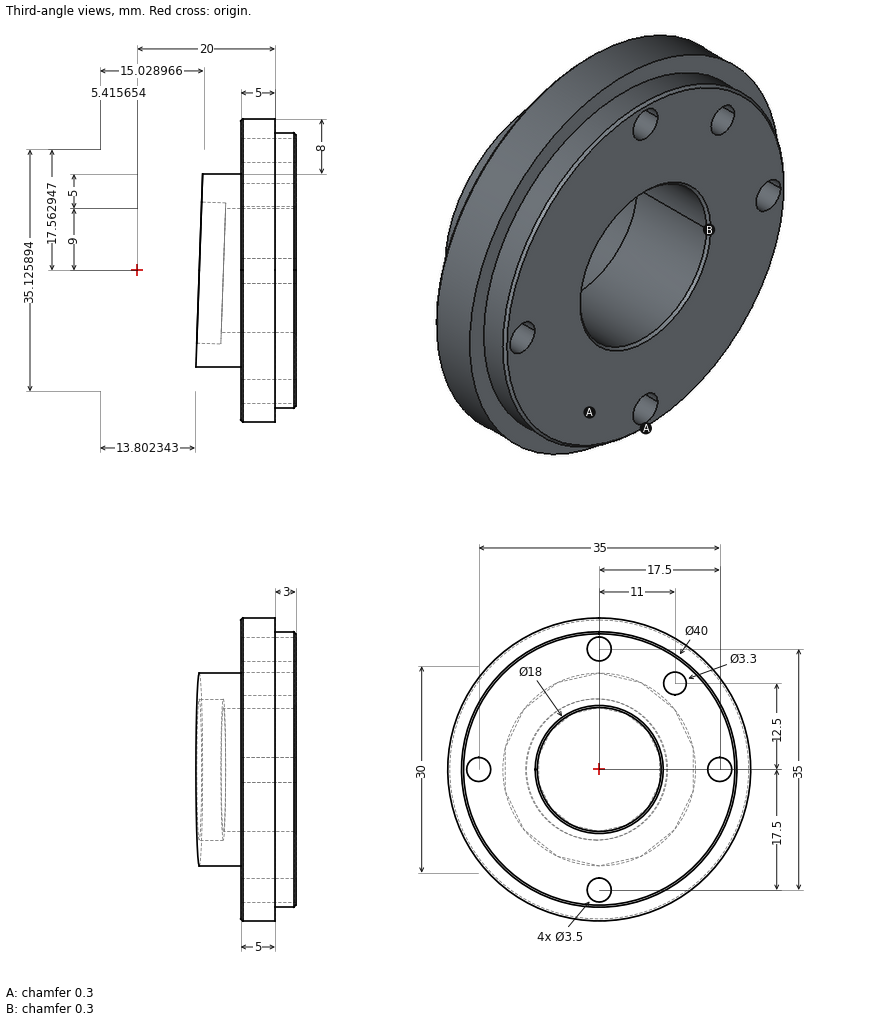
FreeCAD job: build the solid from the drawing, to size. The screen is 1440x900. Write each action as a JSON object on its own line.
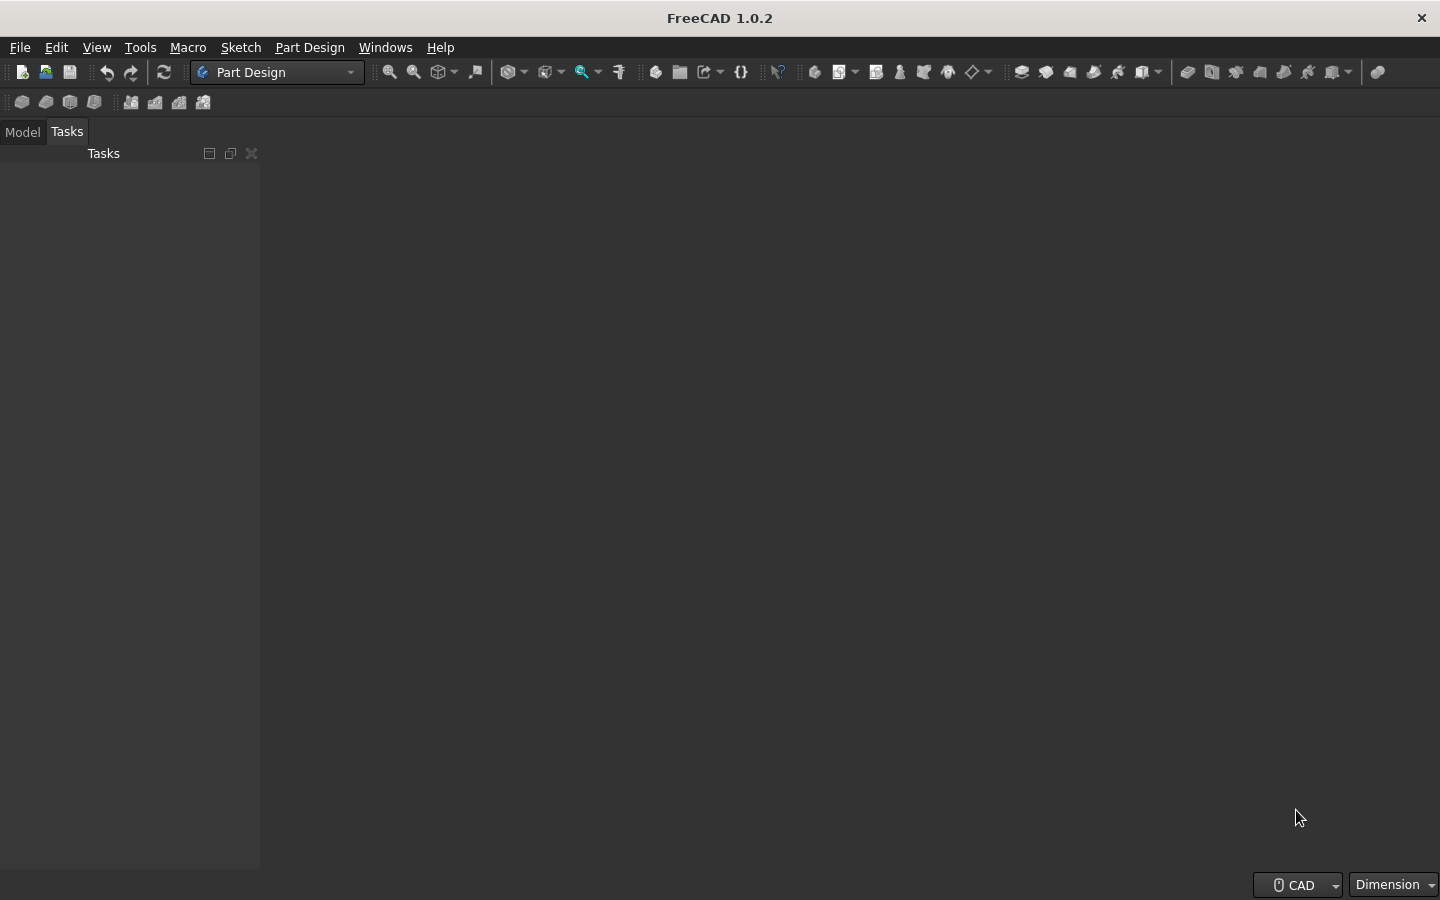
{"action": "left_click", "coordinate": [22, 72]}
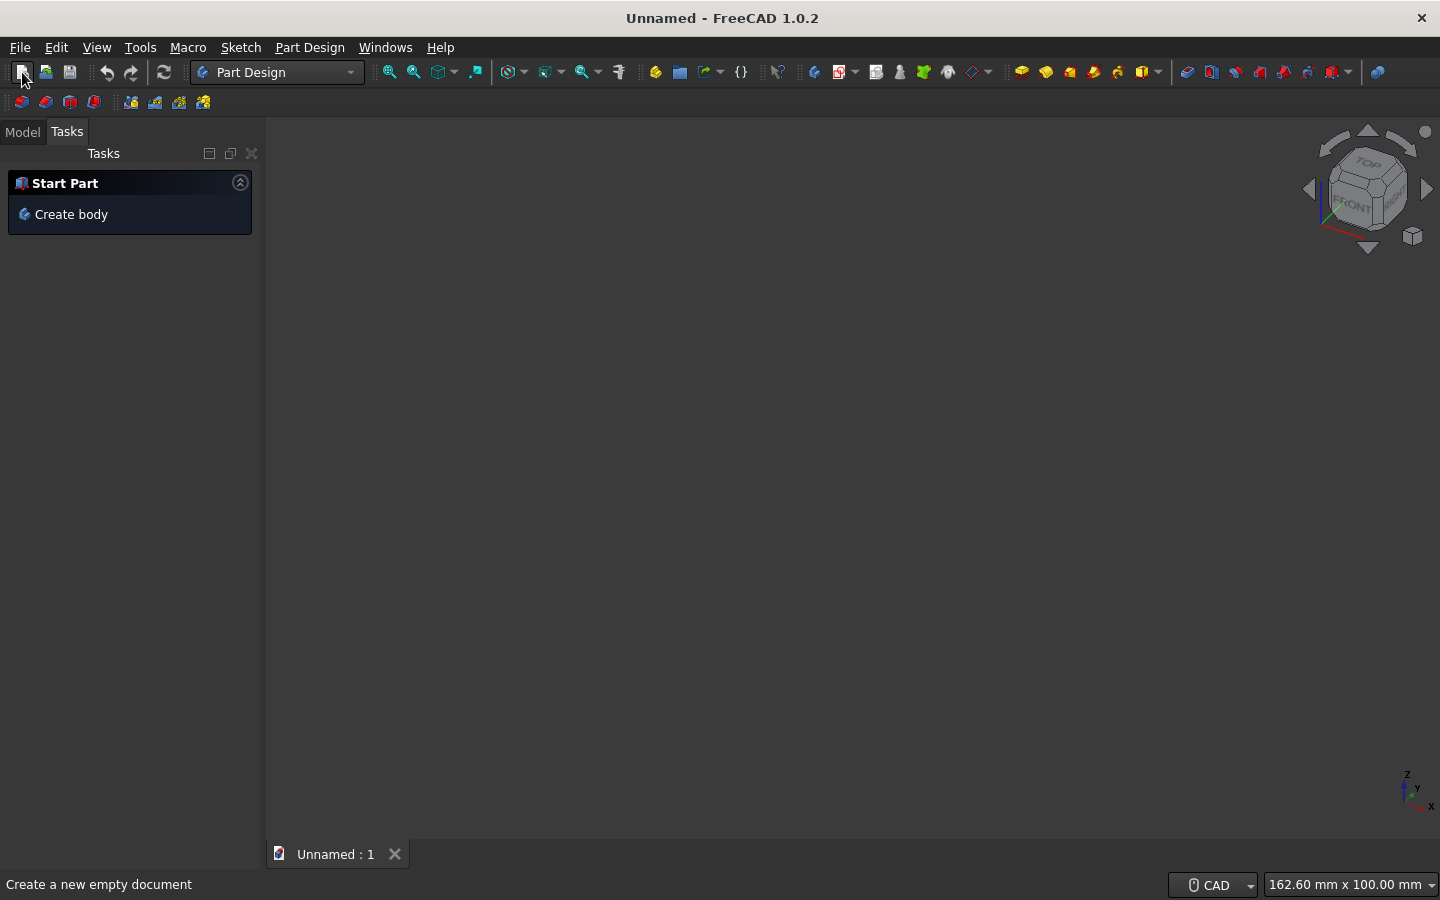
{"action": "left_click", "coordinate": [840, 72]}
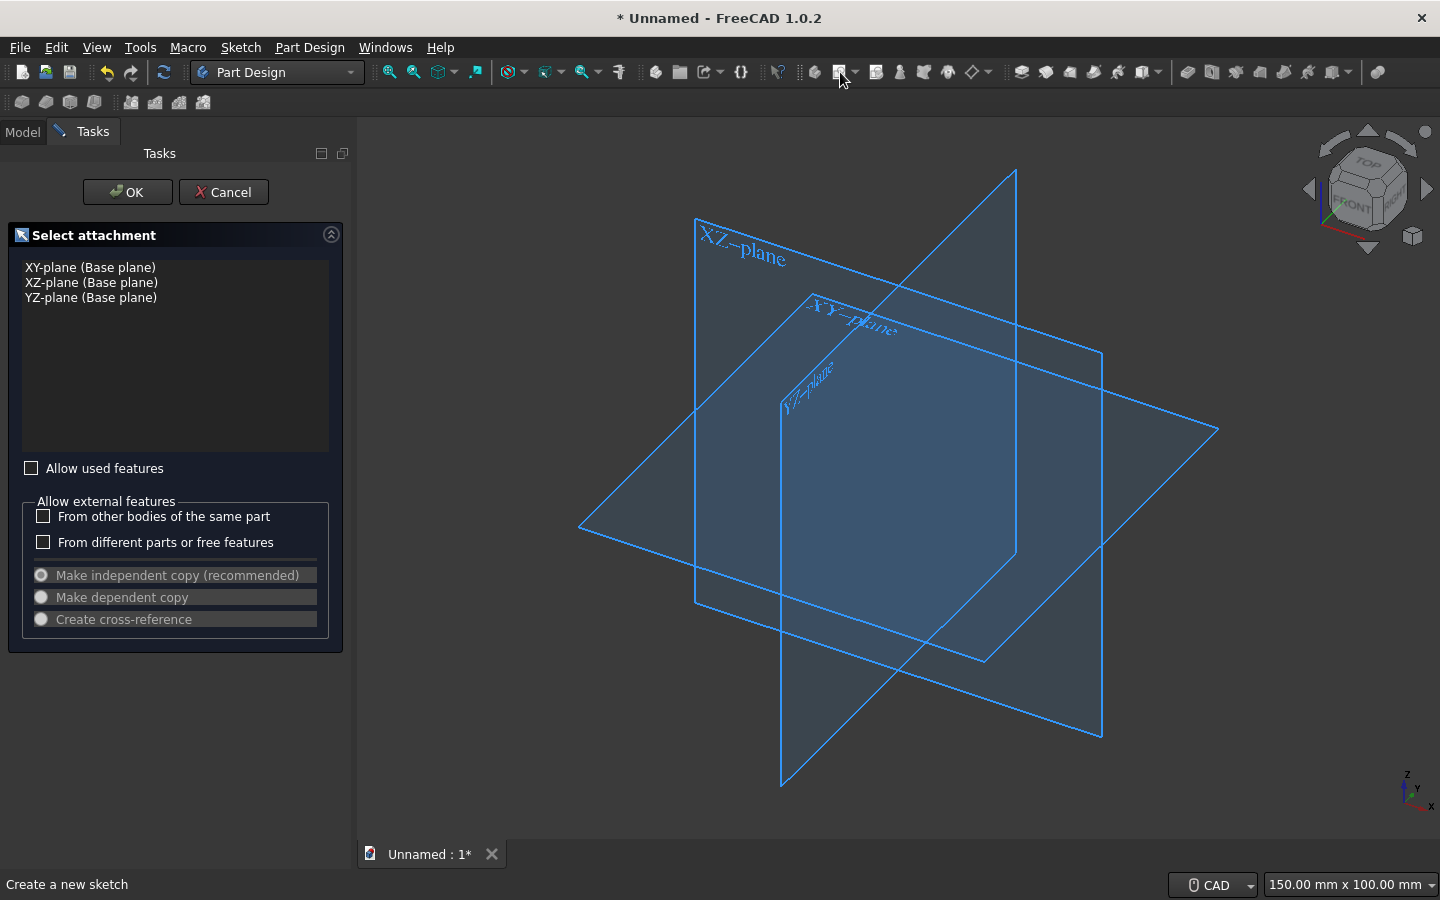
{"action": "left_click", "coordinate": [82, 268]}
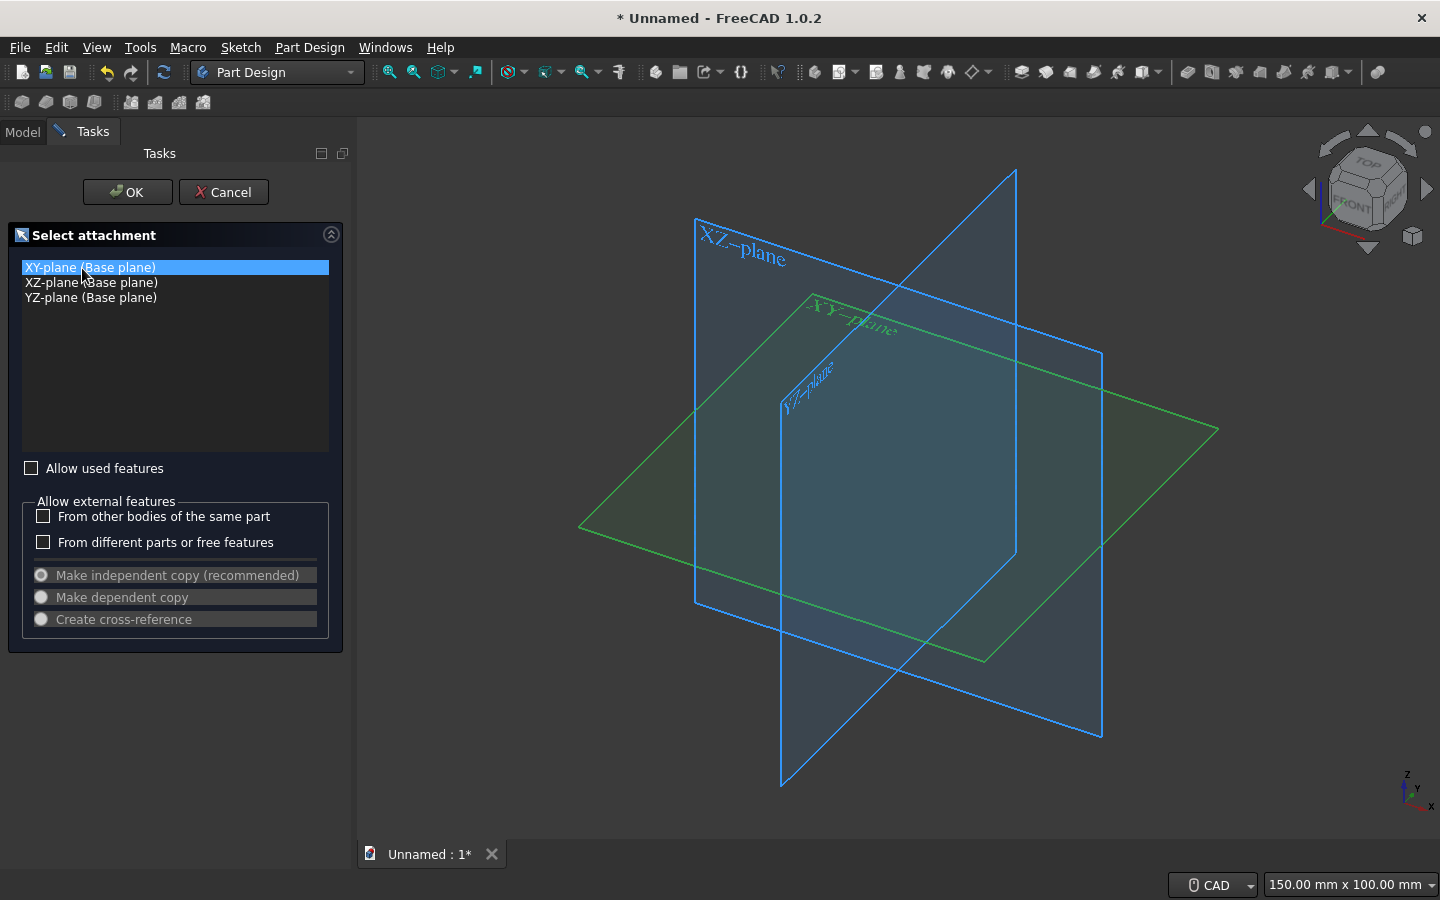
{"action": "left_click", "coordinate": [128, 192]}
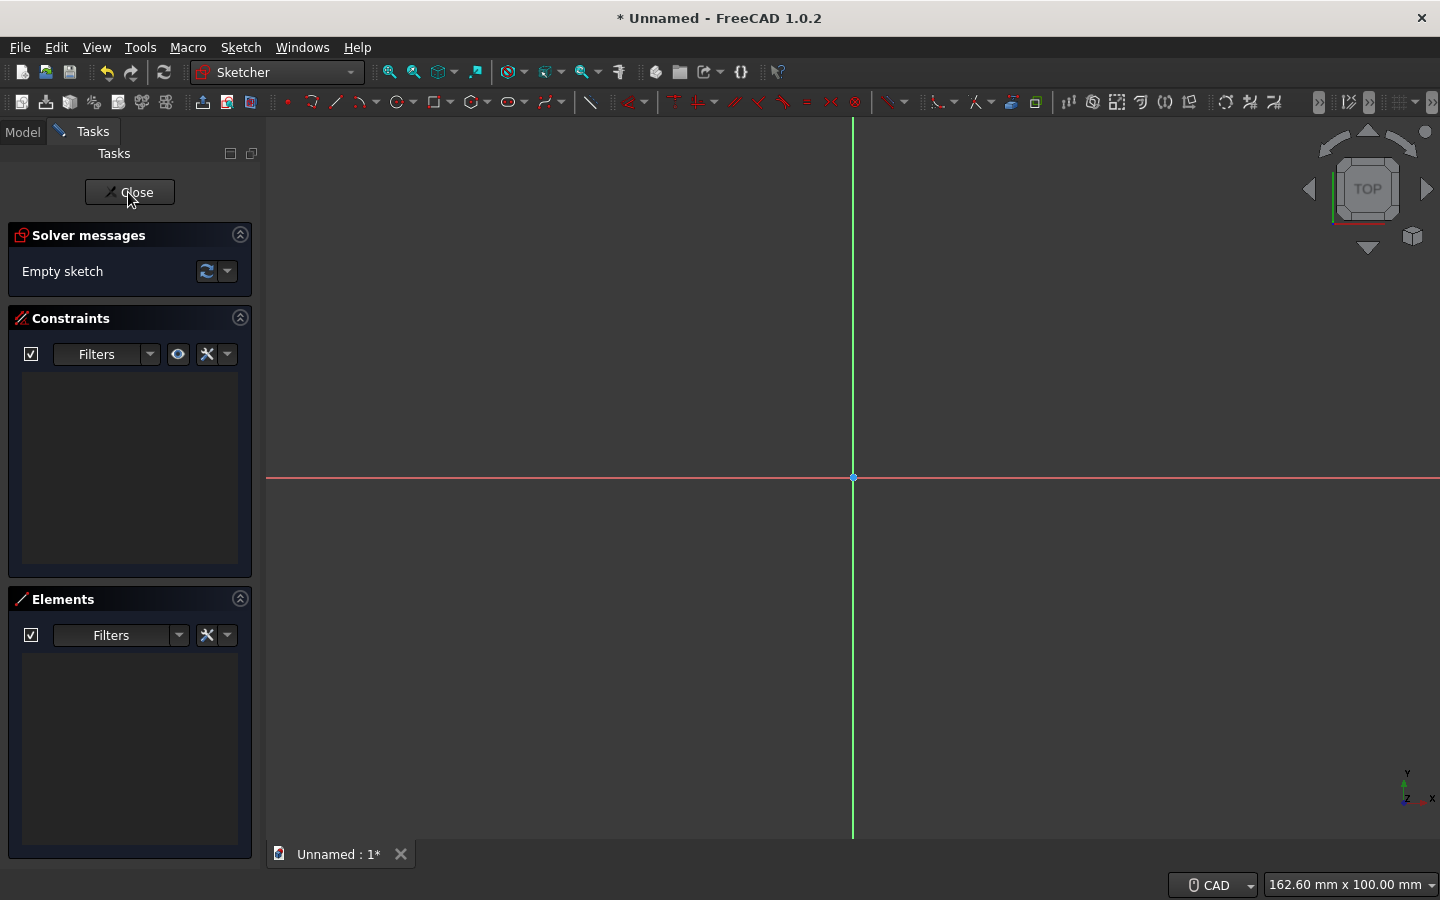
{"action": "scroll", "coordinate": [1007, 352], "scroll_direction": "up", "scroll_amount": 5}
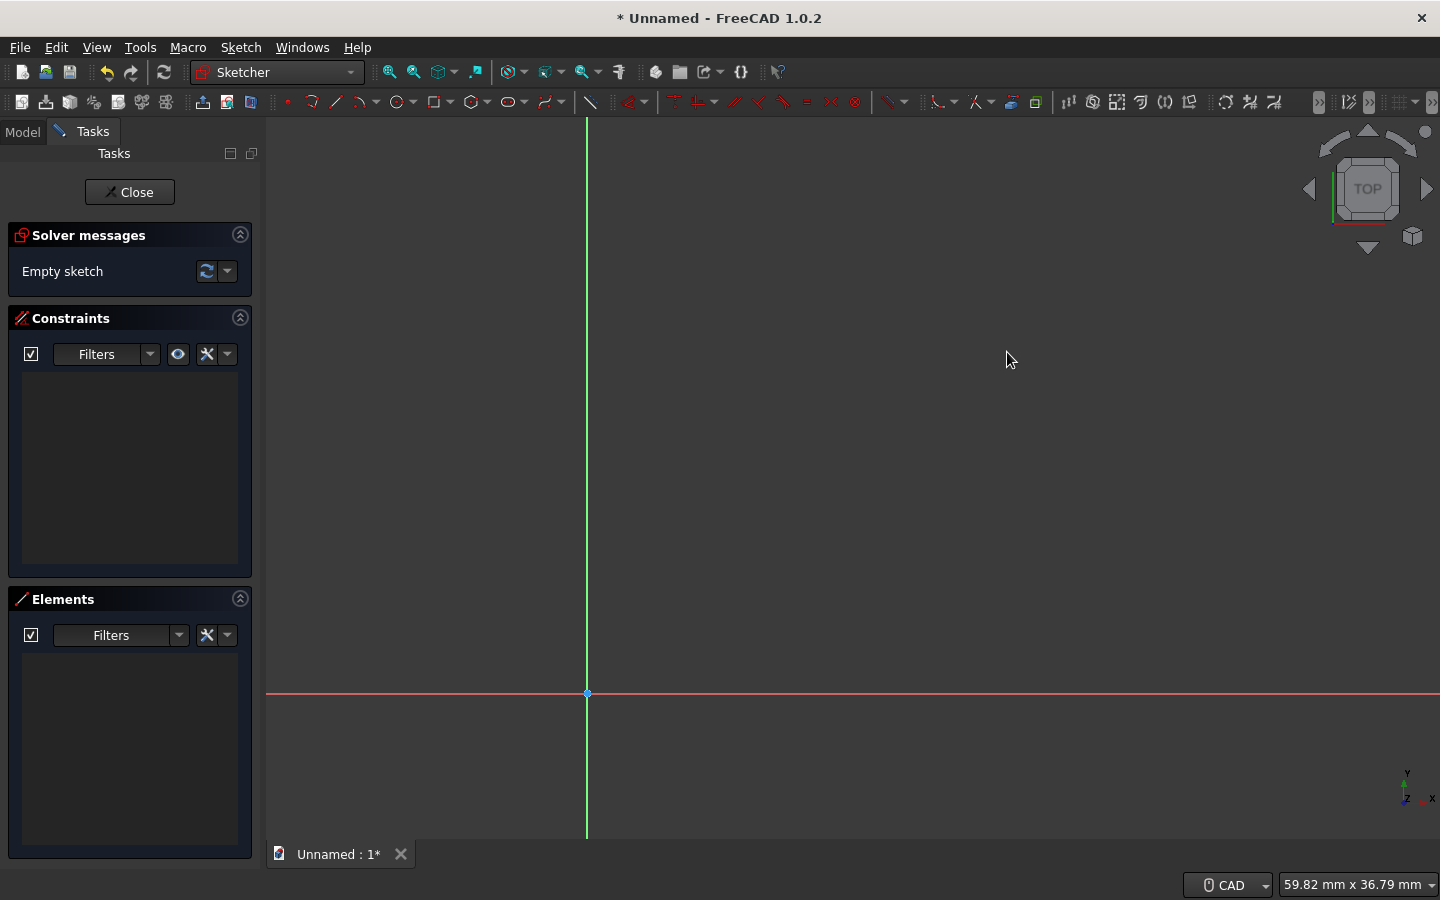
{"action": "left_click", "coordinate": [312, 102]}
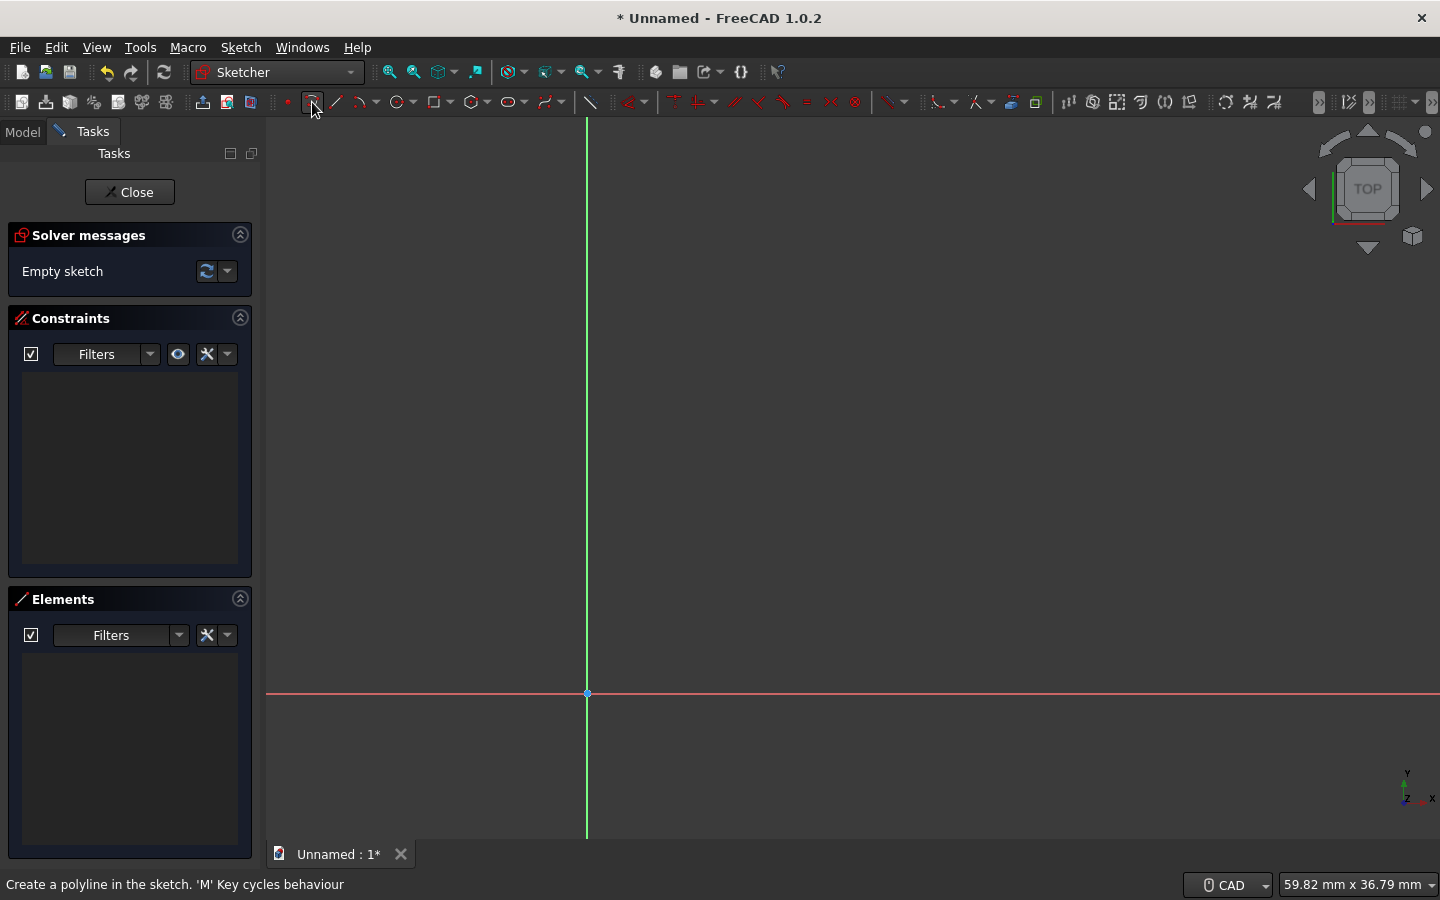
{"action": "left_click", "coordinate": [587, 517]}
{"action": "left_click", "coordinate": [980, 517]}
{"action": "left_click", "coordinate": [980, 262]}
{"action": "left_click", "coordinate": [882, 262]}
{"action": "left_click", "coordinate": [882, 419]}
{"action": "left_click", "coordinate": [596, 419]}
{"action": "left_click", "coordinate": [587, 518]}
{"action": "key", "text": "Escape"}
{"action": "key", "text": "Escape"}